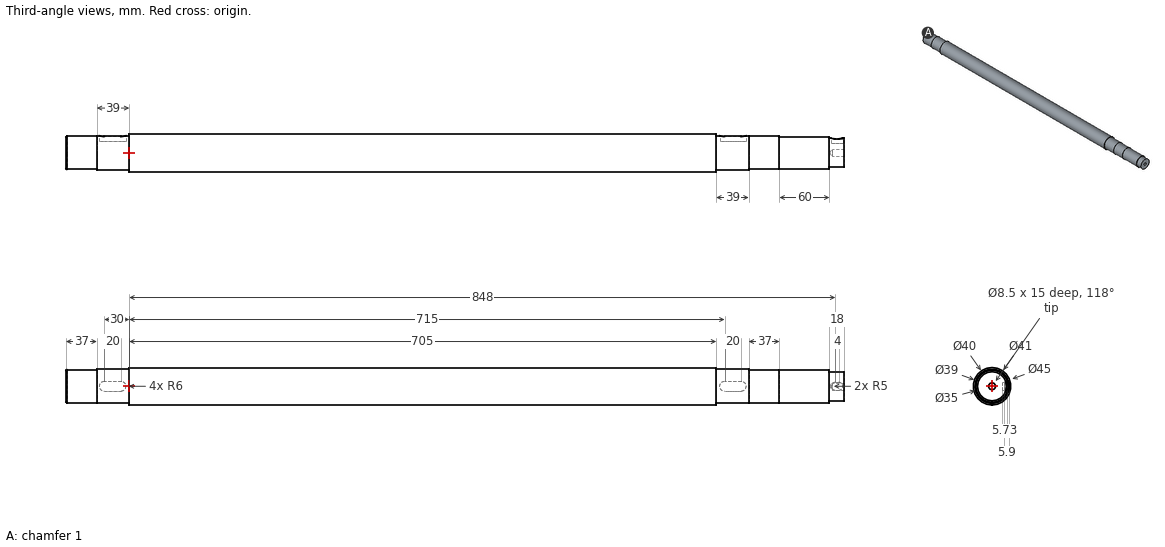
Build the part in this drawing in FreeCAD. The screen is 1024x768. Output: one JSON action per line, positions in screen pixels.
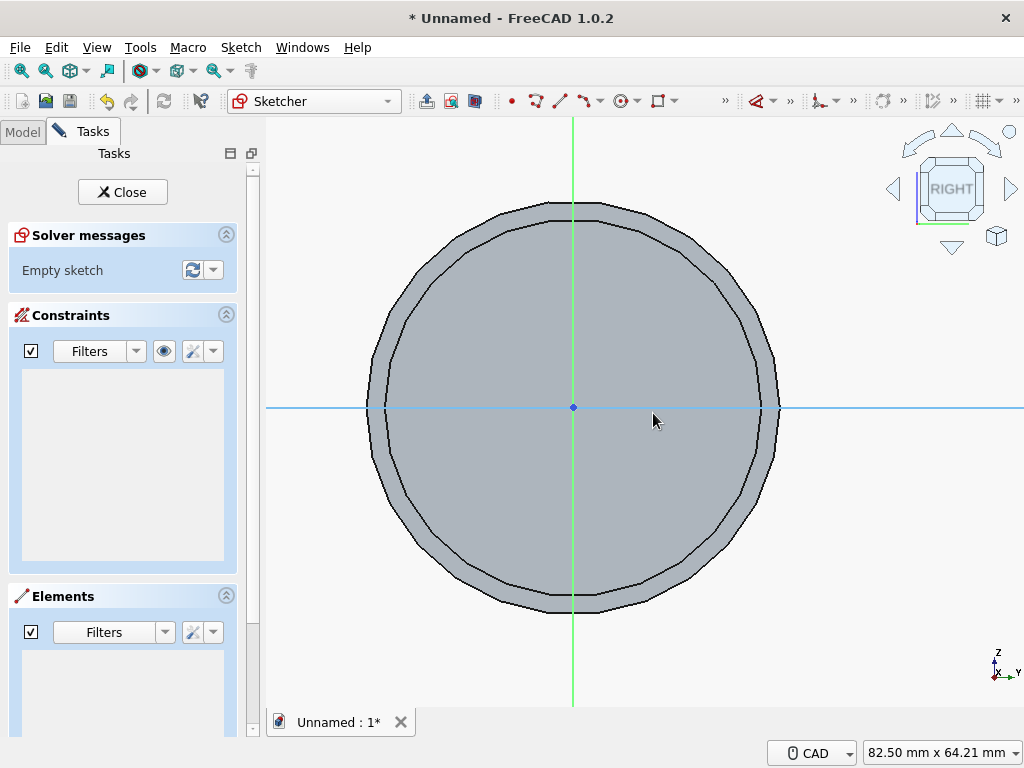
{"action": "left_click", "coordinate": [622, 102]}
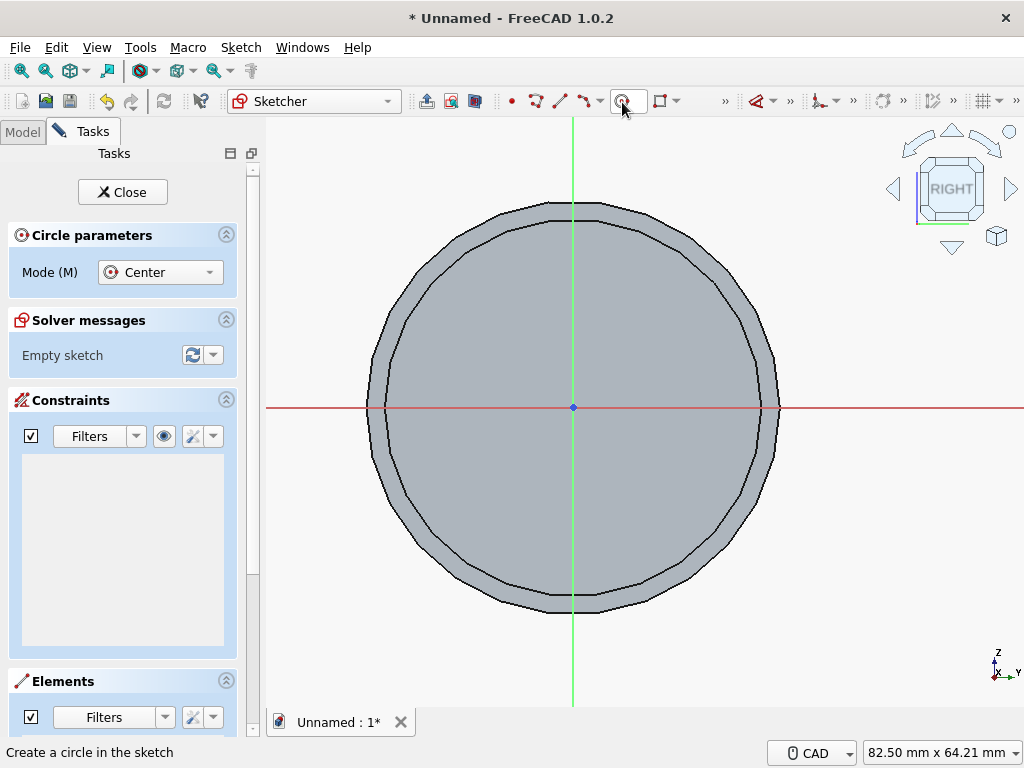
{"action": "left_click", "coordinate": [573, 408]}
{"action": "mouse_move", "coordinate": [703, 278]}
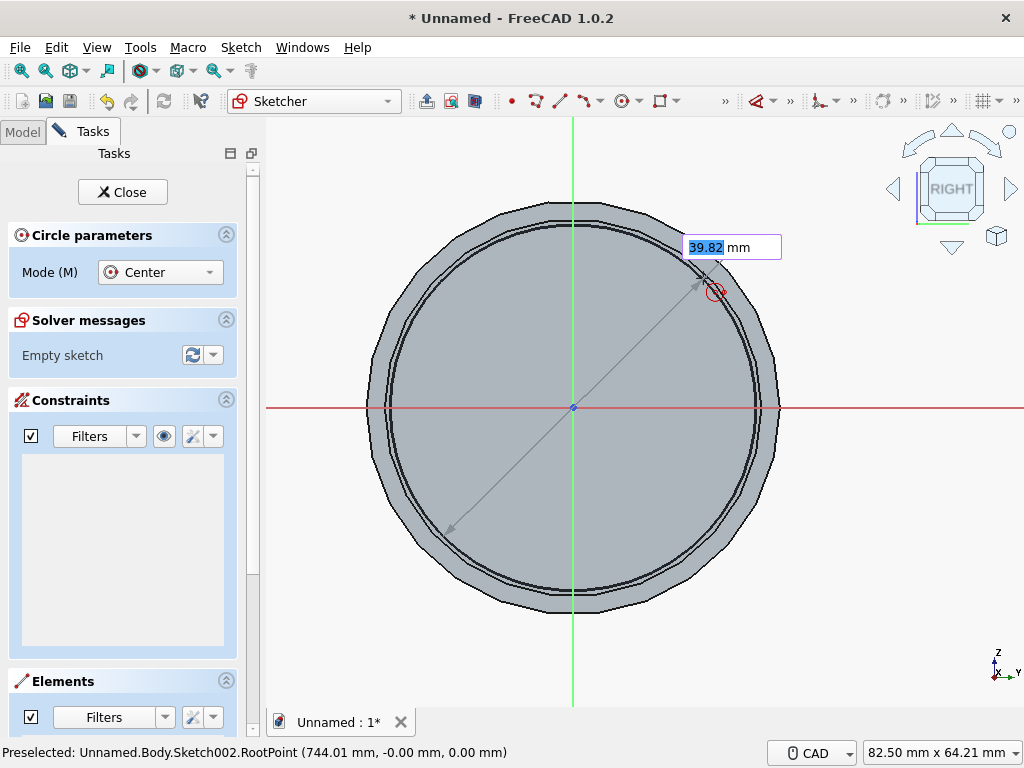
{"action": "type", "text": "40"}
{"action": "key", "text": "Return"}
{"action": "key", "text": "Escape"}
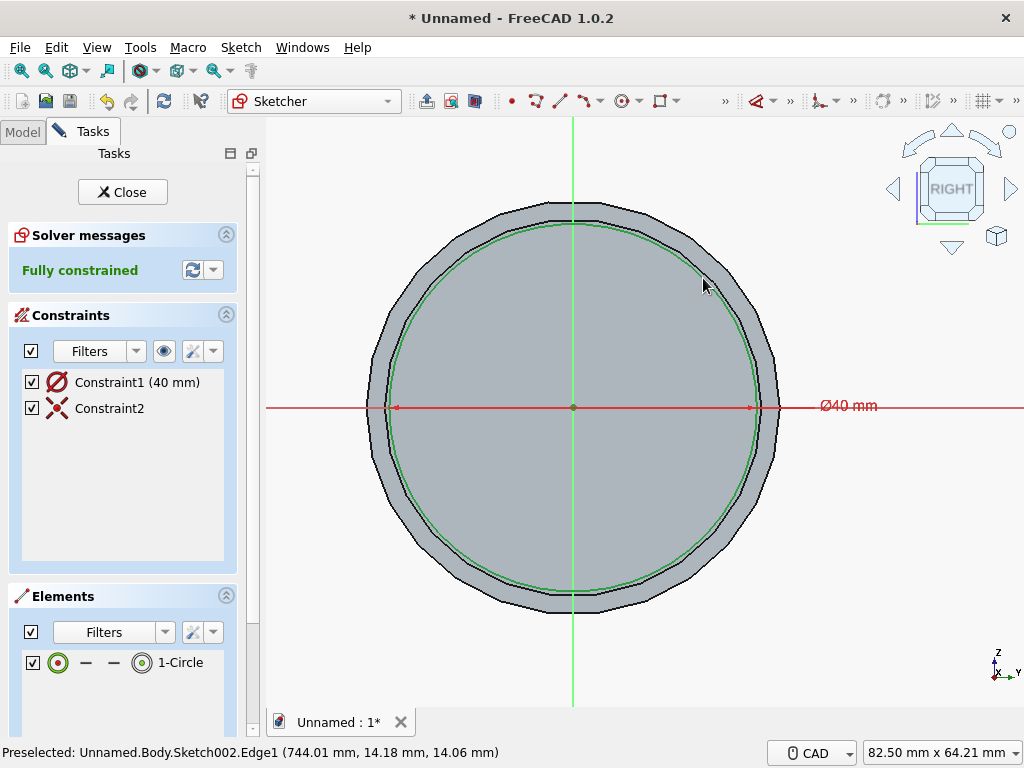
{"action": "left_click", "coordinate": [123, 192]}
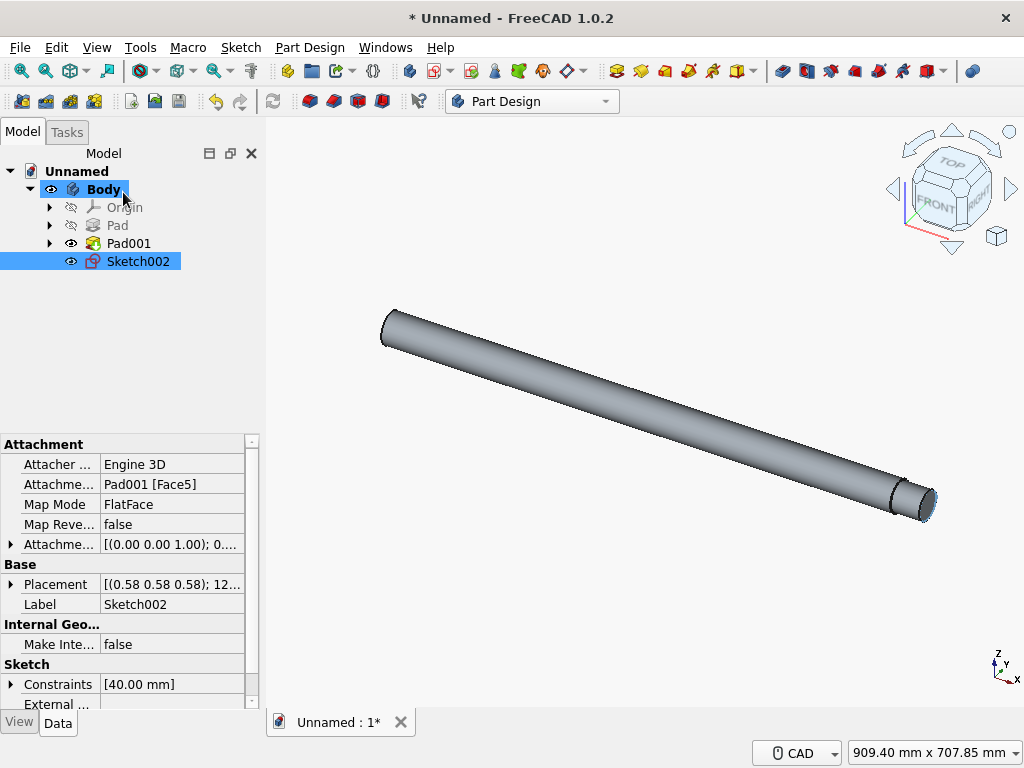
{"action": "left_click", "coordinate": [618, 72]}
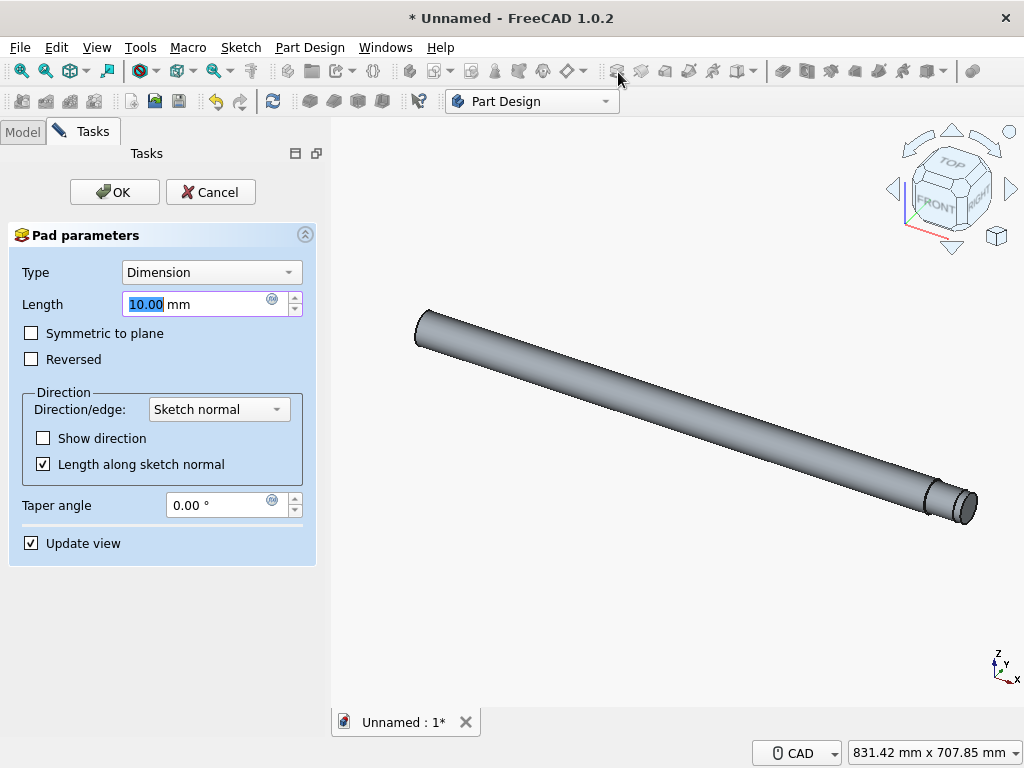
{"action": "type", "text": "37"}
{"action": "key", "text": "Tab"}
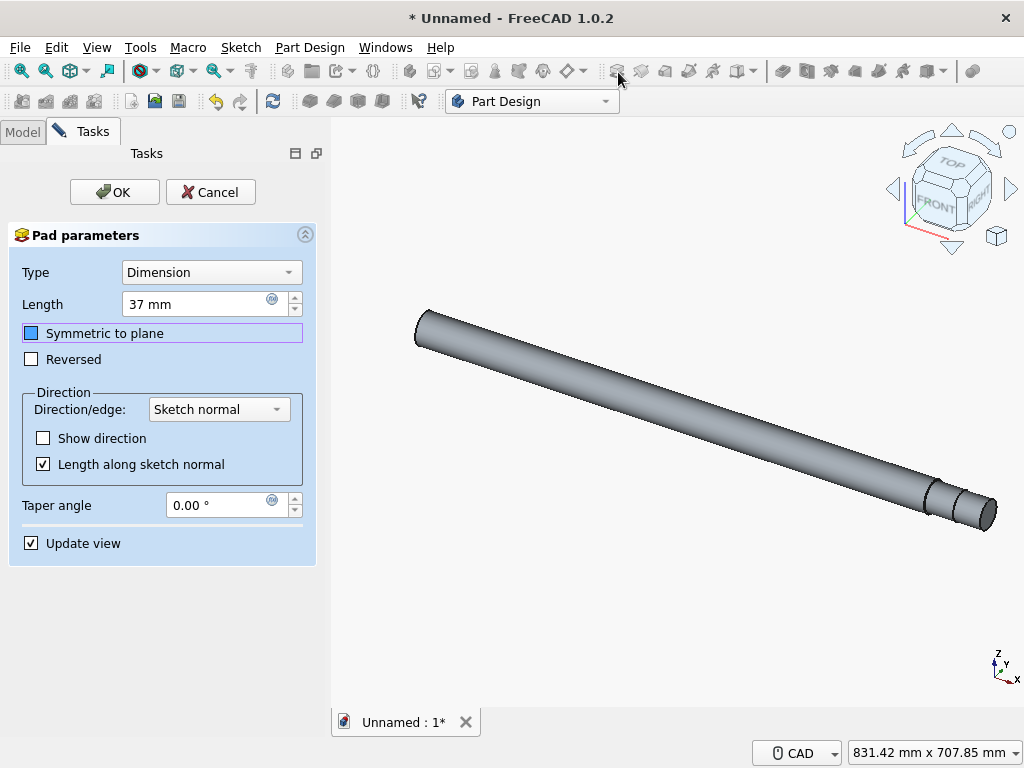
{"action": "left_click", "coordinate": [115, 192]}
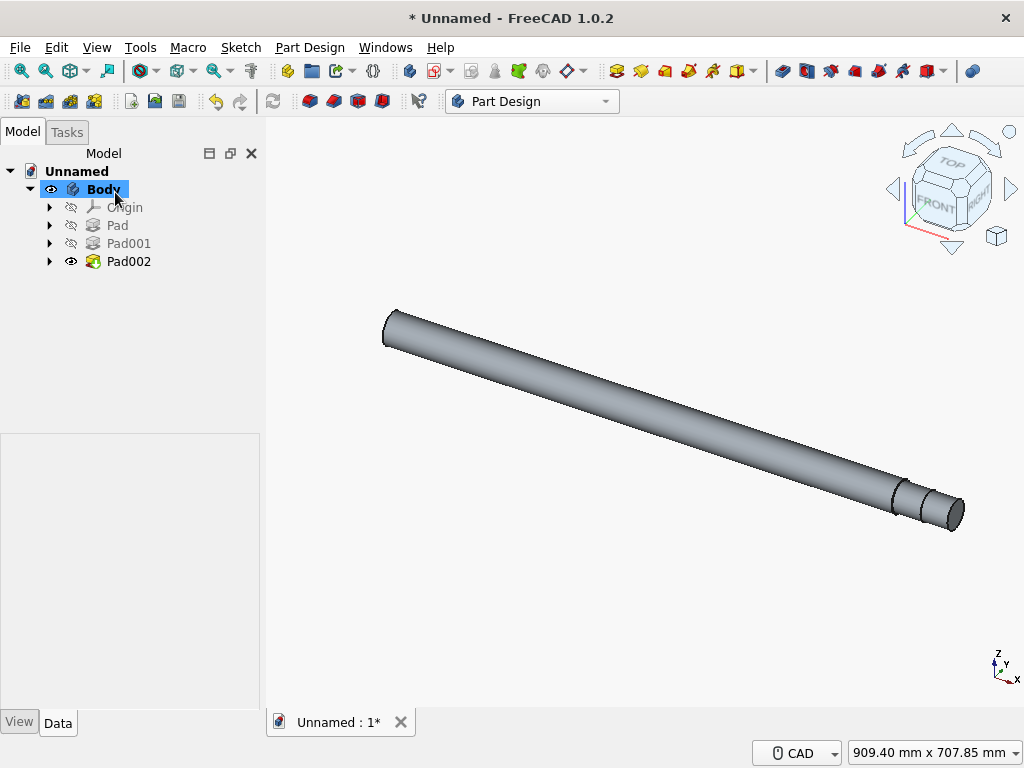
{"action": "left_click", "coordinate": [958, 515]}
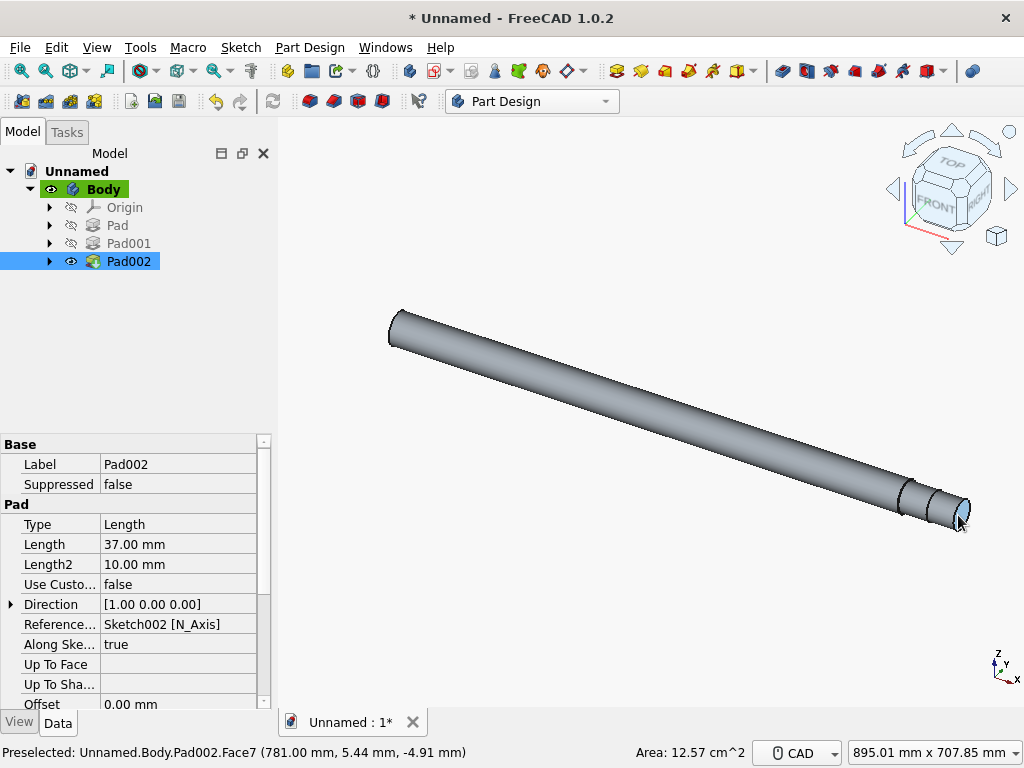
{"action": "left_click", "coordinate": [434, 72]}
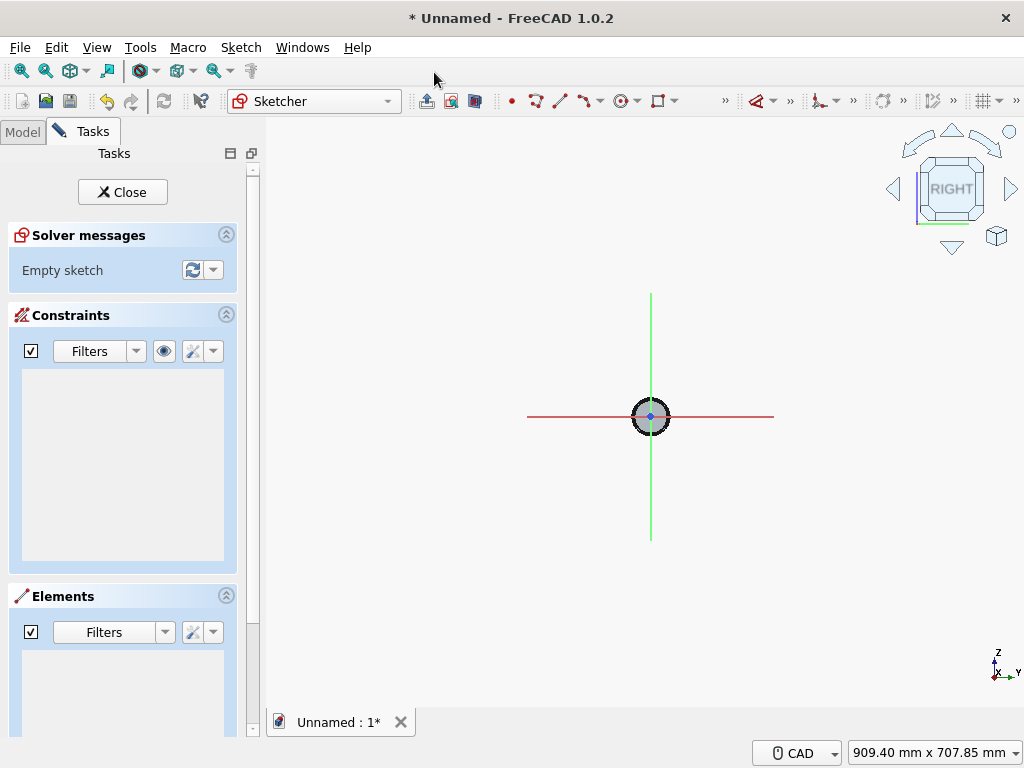
{"action": "scroll", "coordinate": [658, 417], "scroll_direction": "up", "scroll_amount": 12}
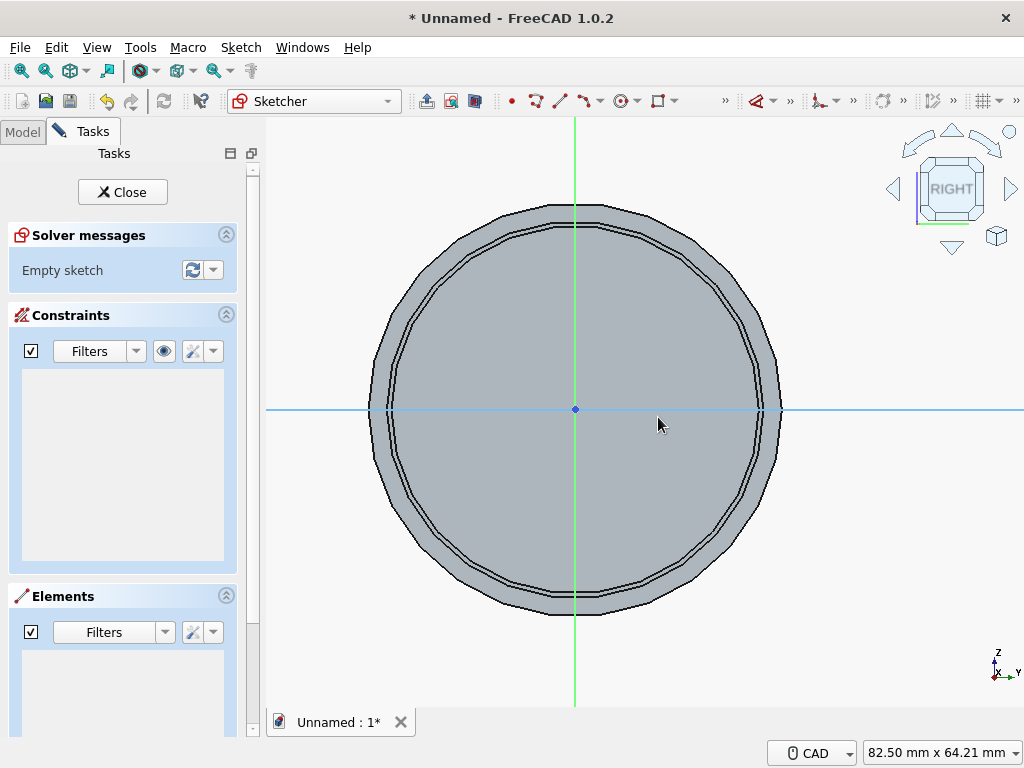
{"action": "left_click", "coordinate": [622, 102]}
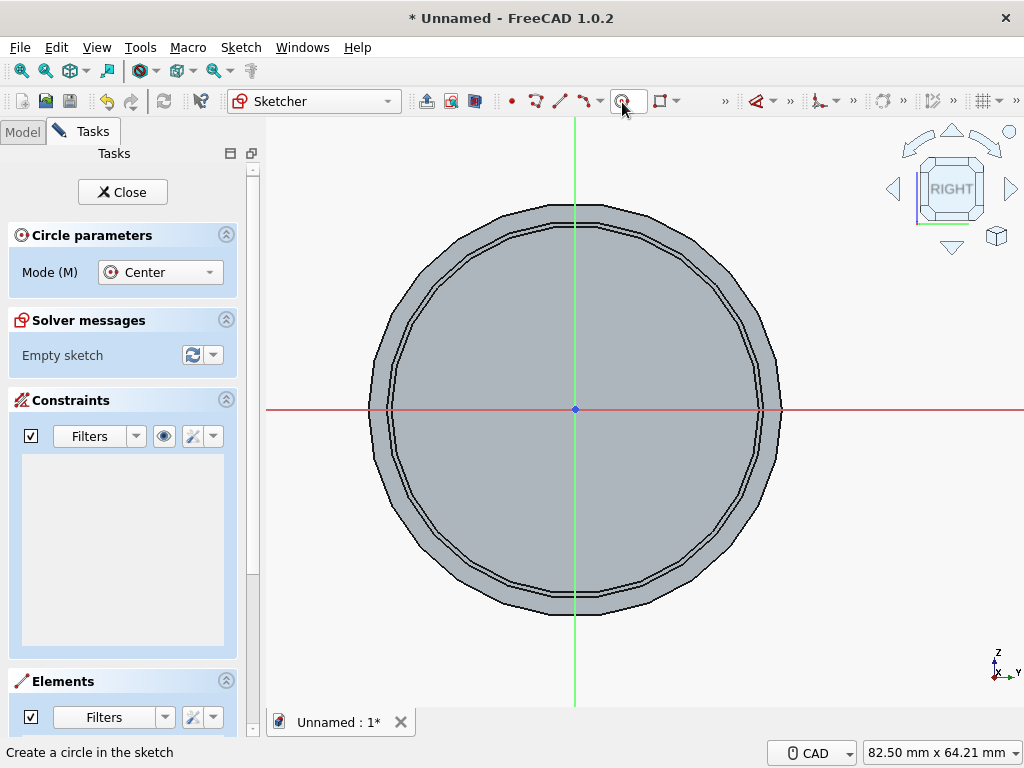
{"action": "left_click", "coordinate": [575, 410]}
{"action": "mouse_move", "coordinate": [702, 283]}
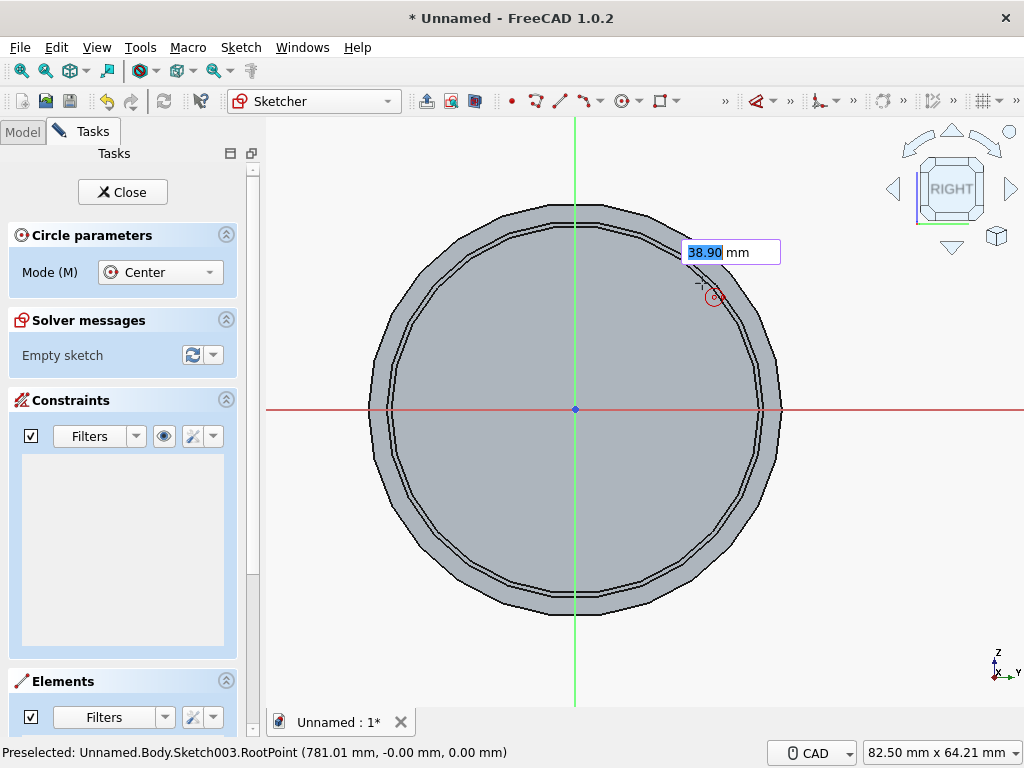
{"action": "type", "text": "39"}
{"action": "key", "text": "Return"}
{"action": "key", "text": "Escape"}